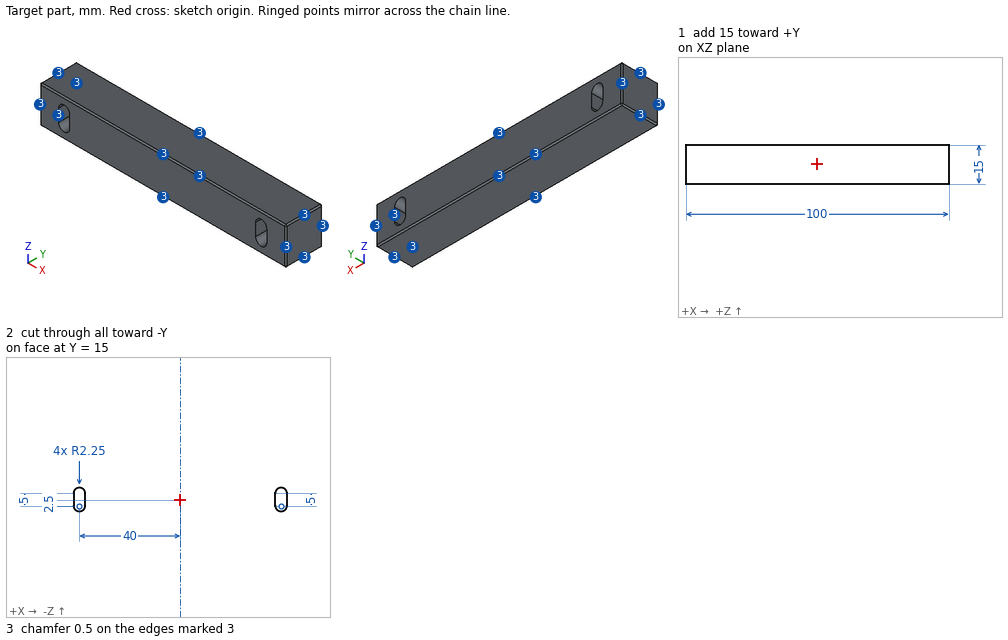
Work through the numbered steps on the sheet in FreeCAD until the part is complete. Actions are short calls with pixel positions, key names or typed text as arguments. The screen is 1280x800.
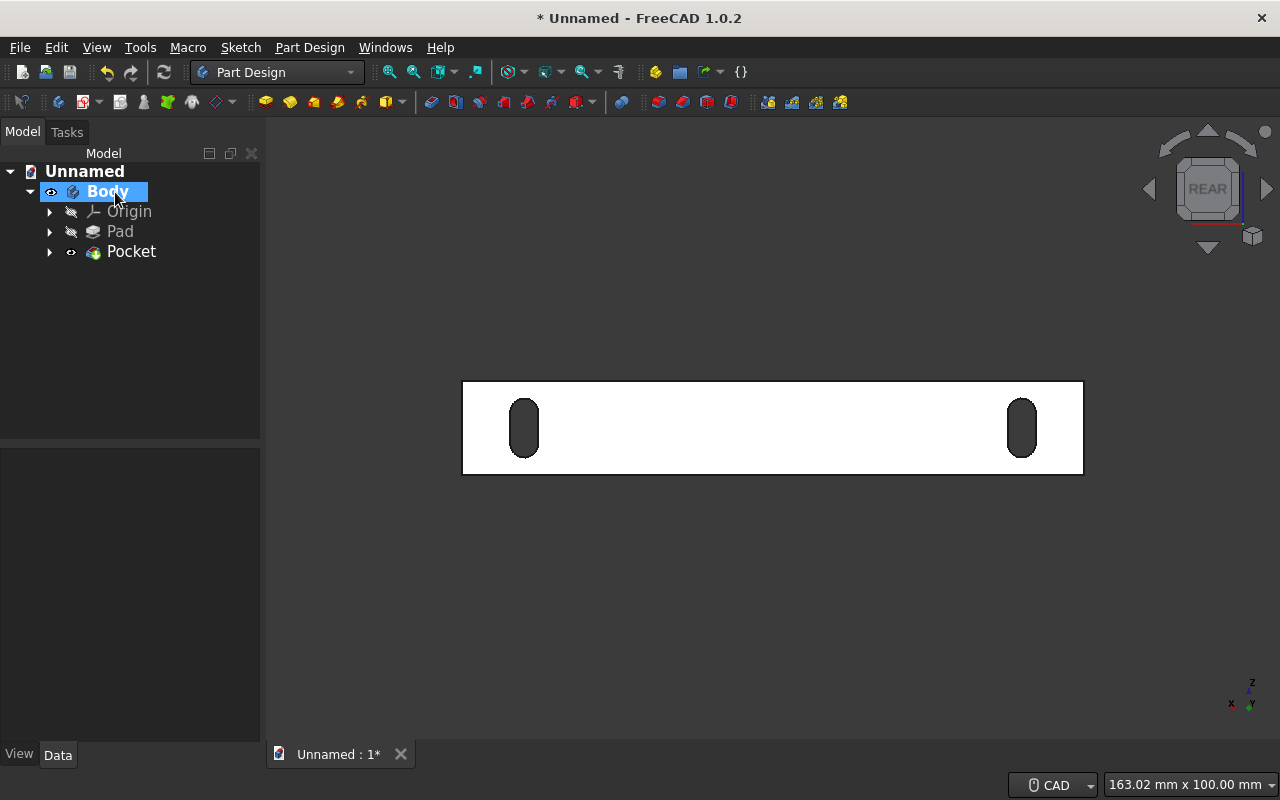
click(1084, 427)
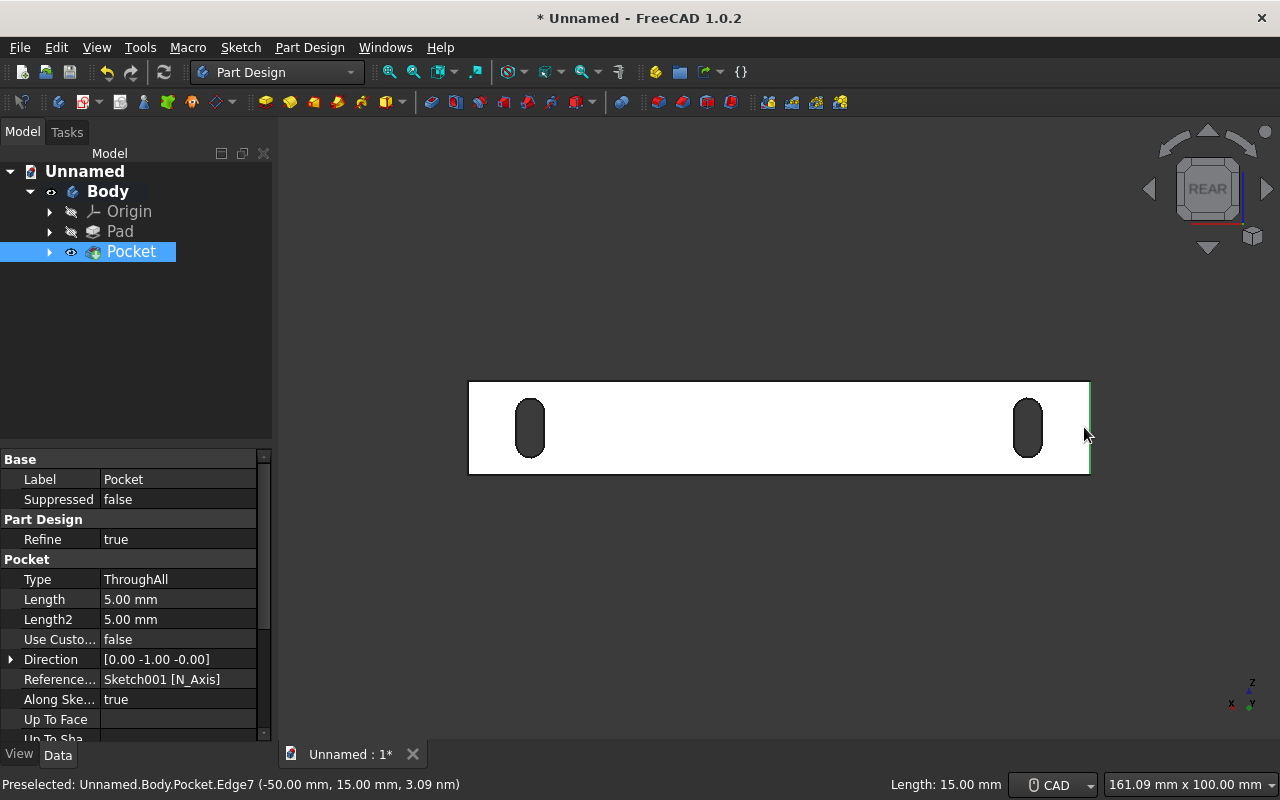
key(0)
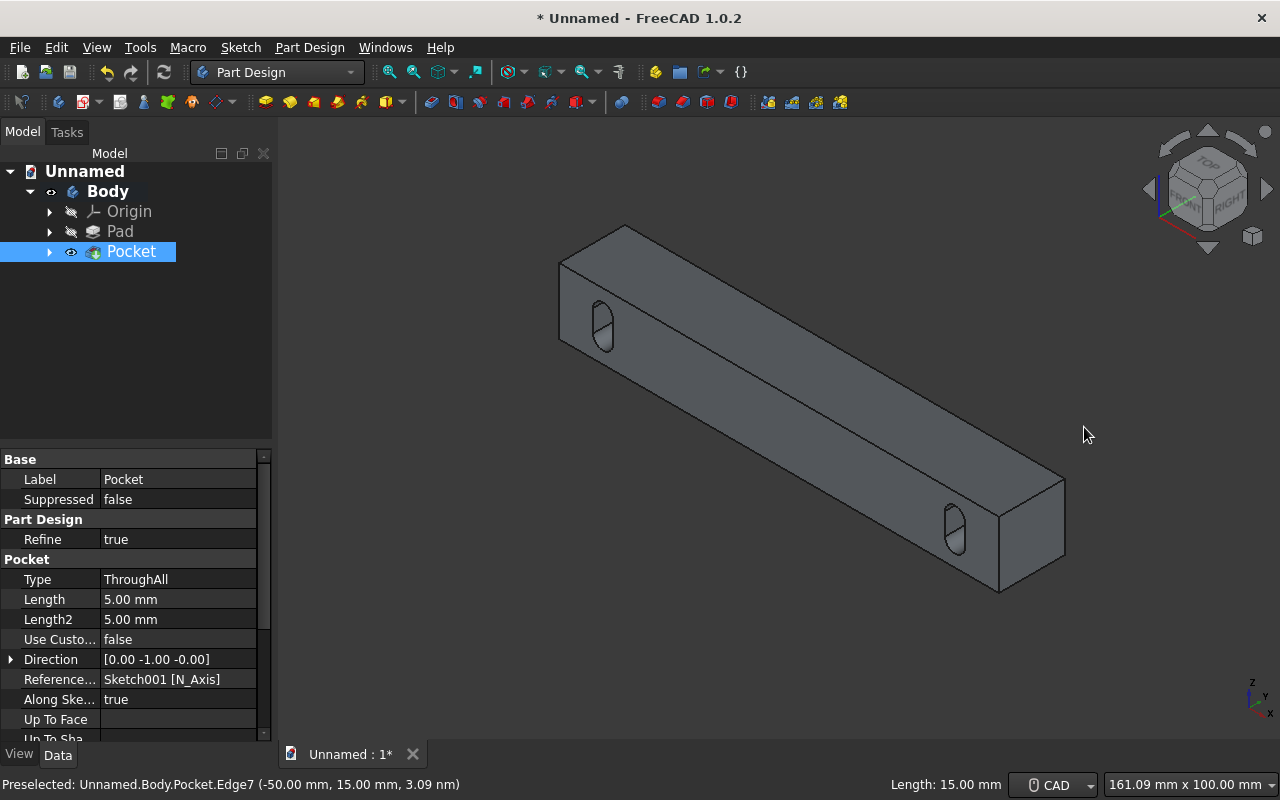
click(938, 442, ctrl)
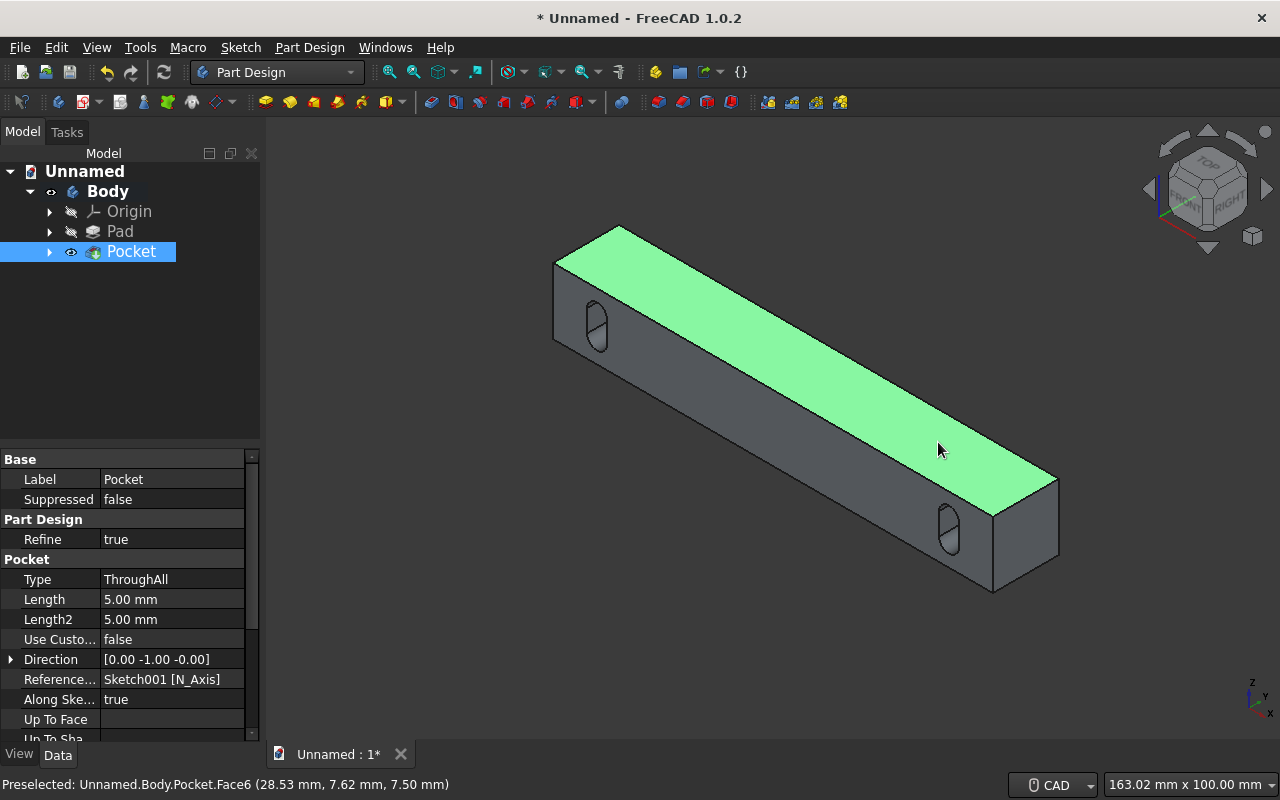
click(993, 554, ctrl)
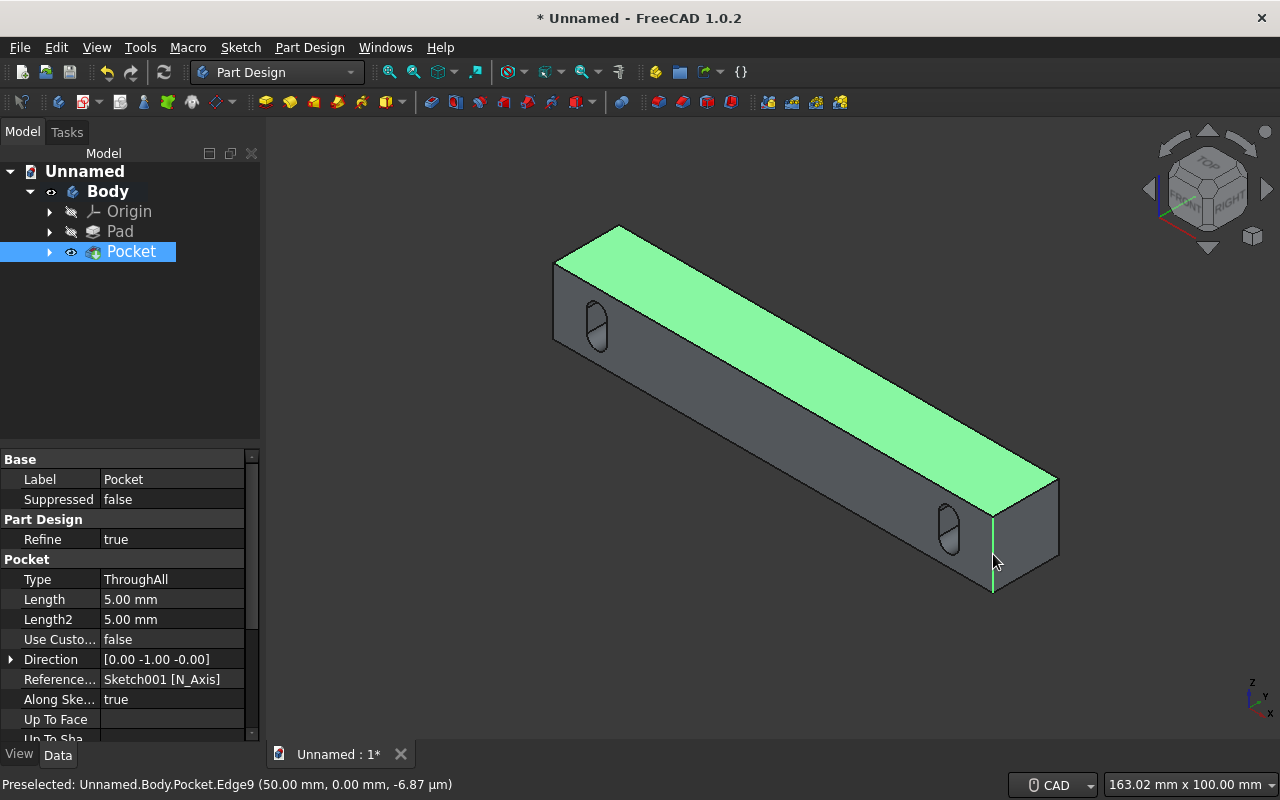
key(2)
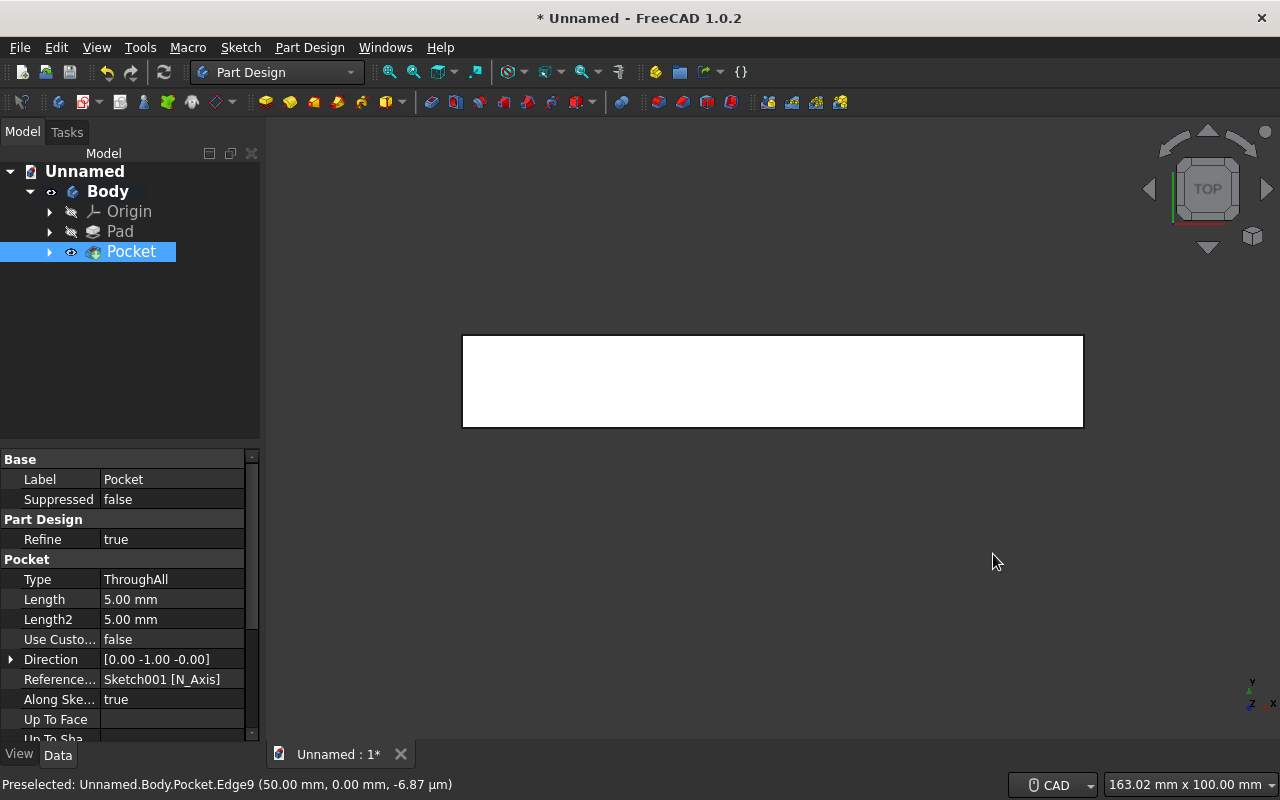
key(1)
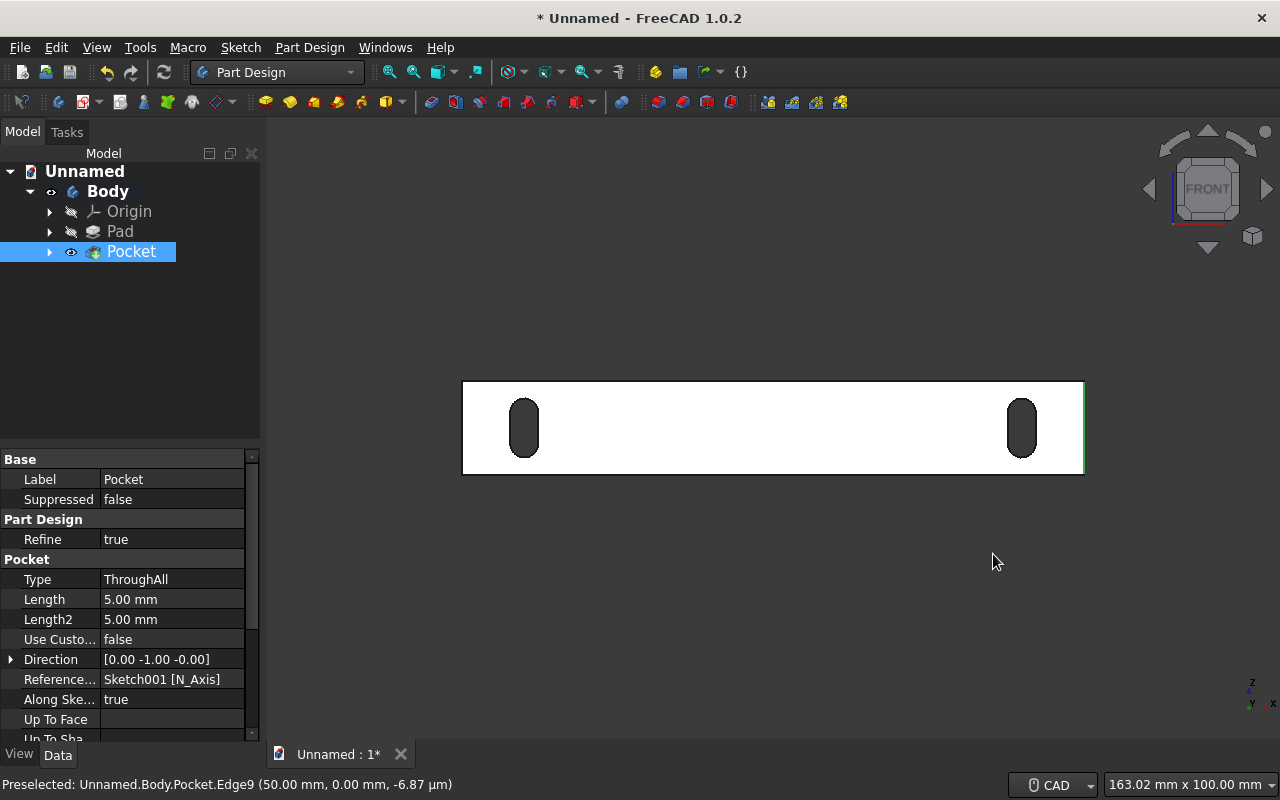
key(3)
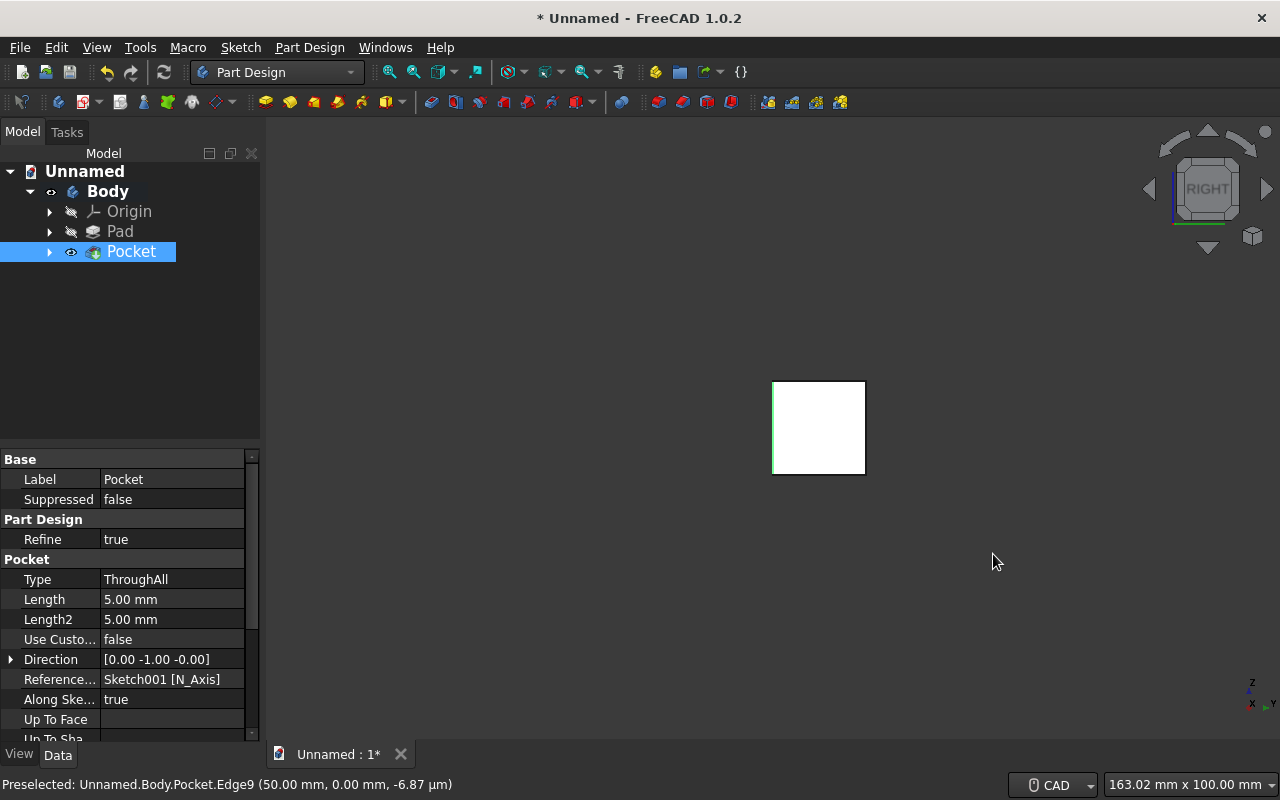
click(390, 72)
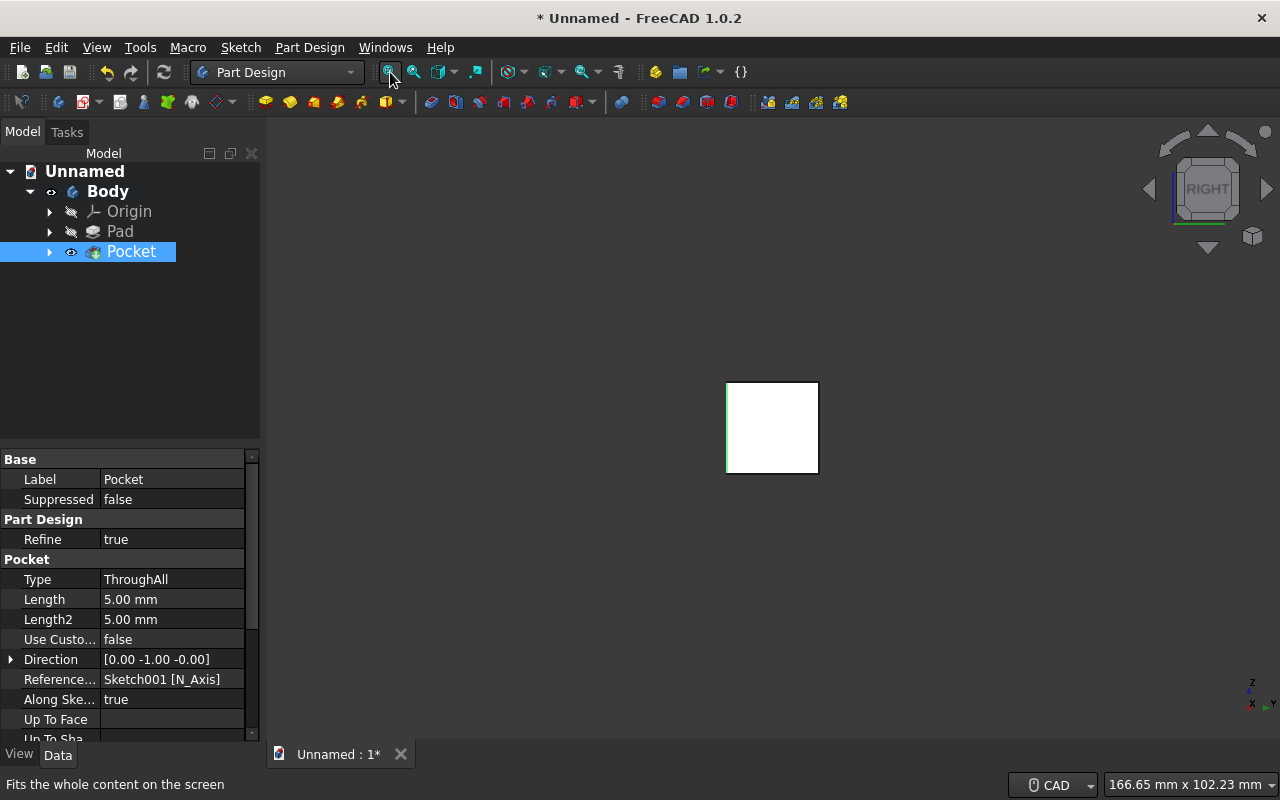
click(819, 427, ctrl)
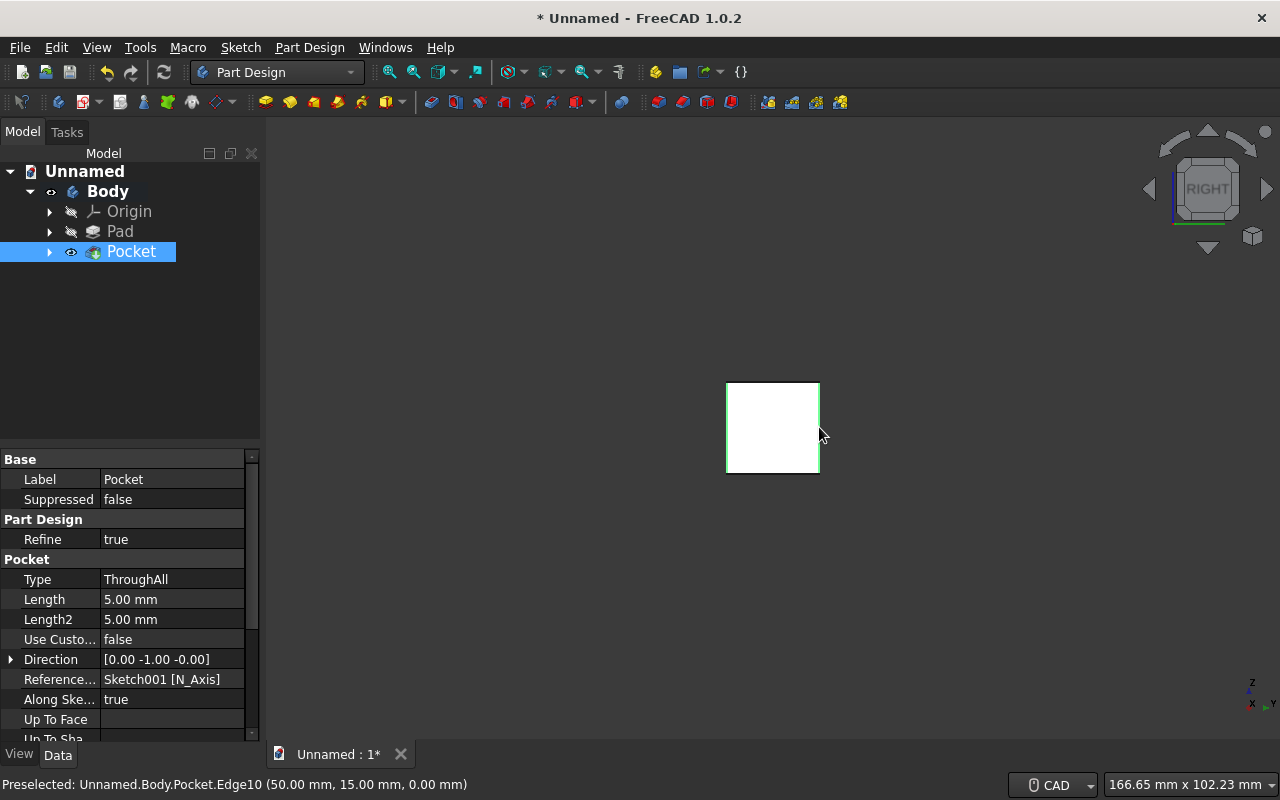
key(5)